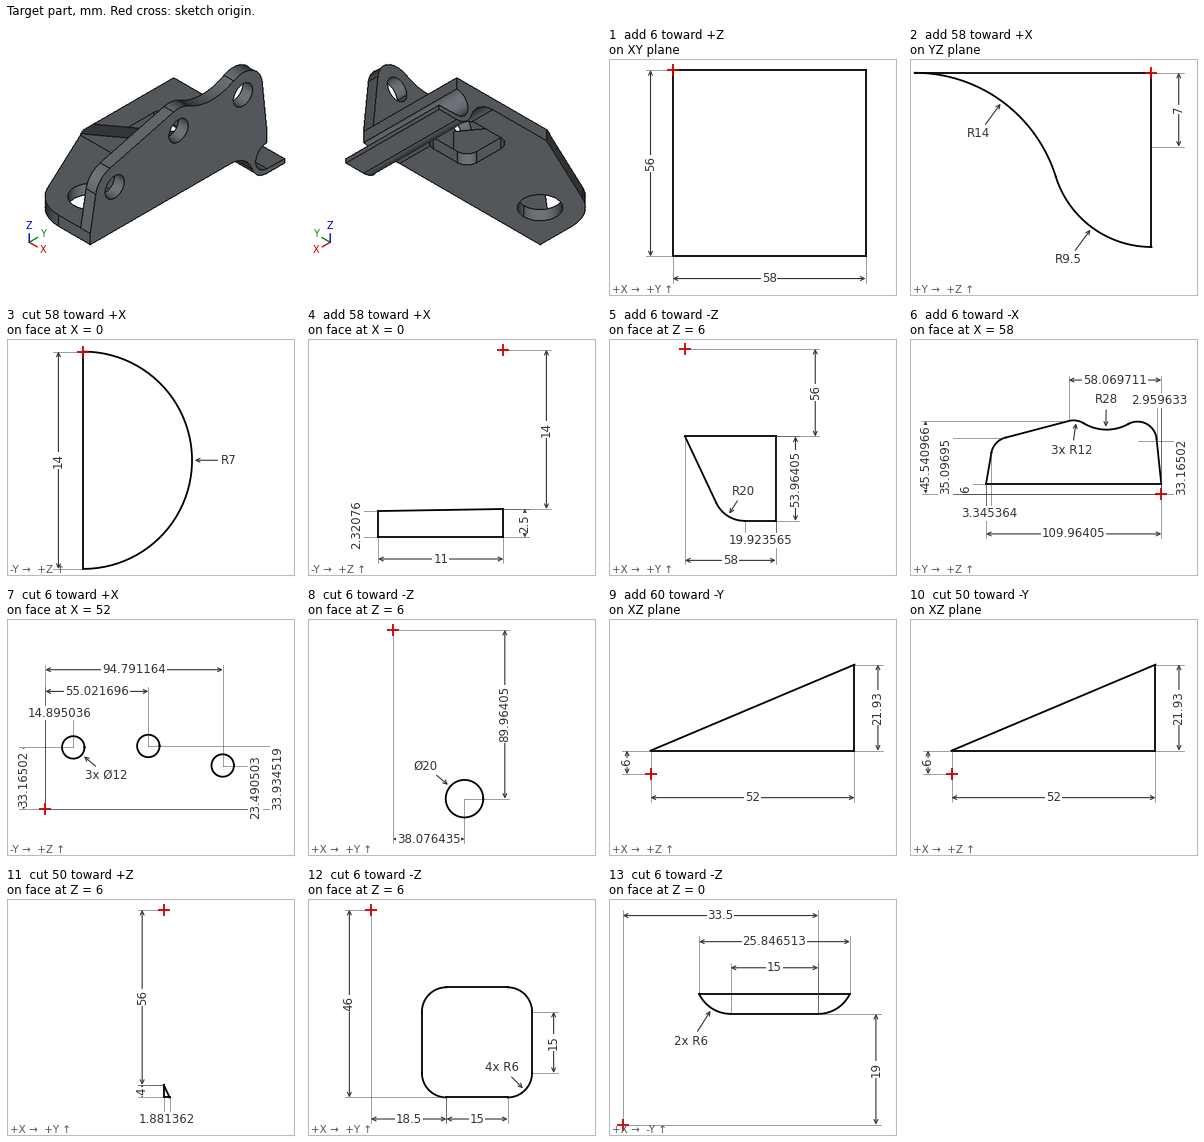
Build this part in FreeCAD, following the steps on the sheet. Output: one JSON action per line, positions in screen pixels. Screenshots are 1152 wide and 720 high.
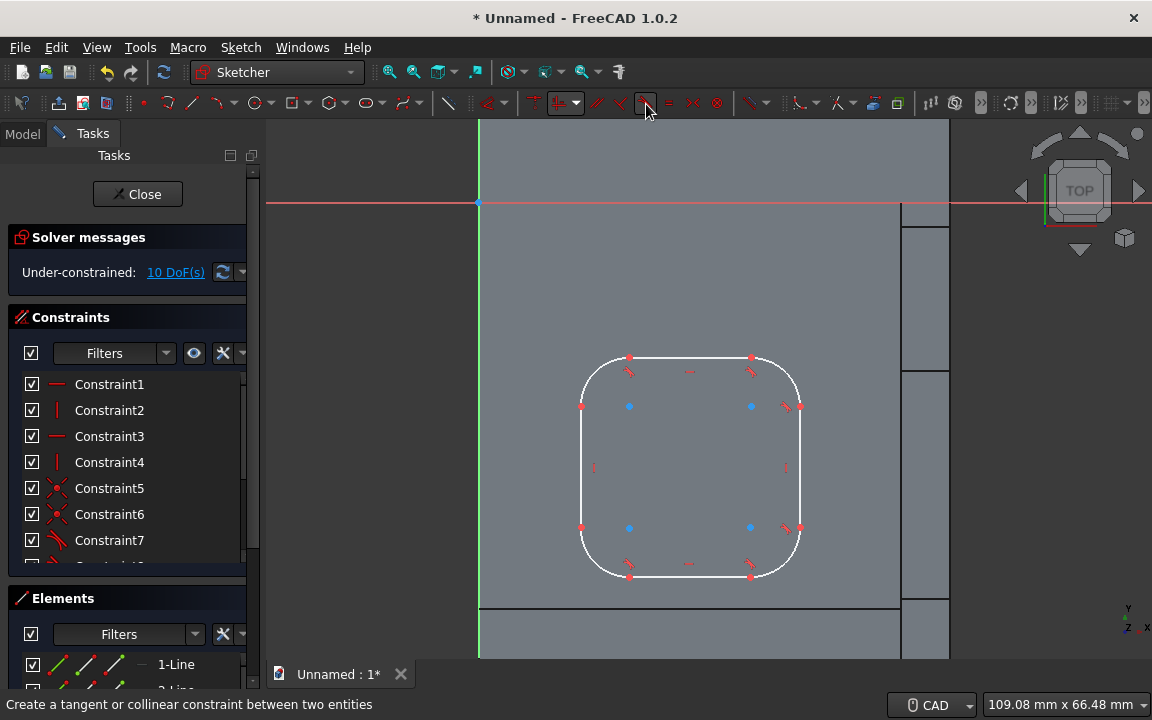
{"action": "left_click", "coordinate": [581, 443]}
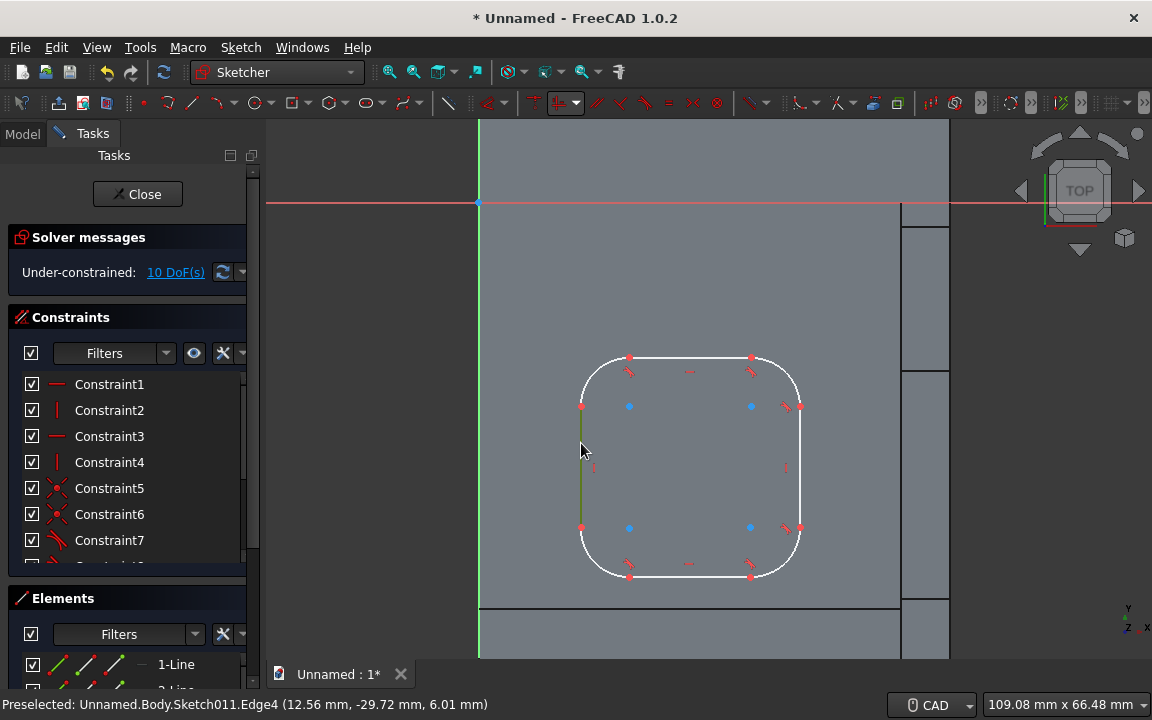
{"action": "left_click", "coordinate": [607, 363]}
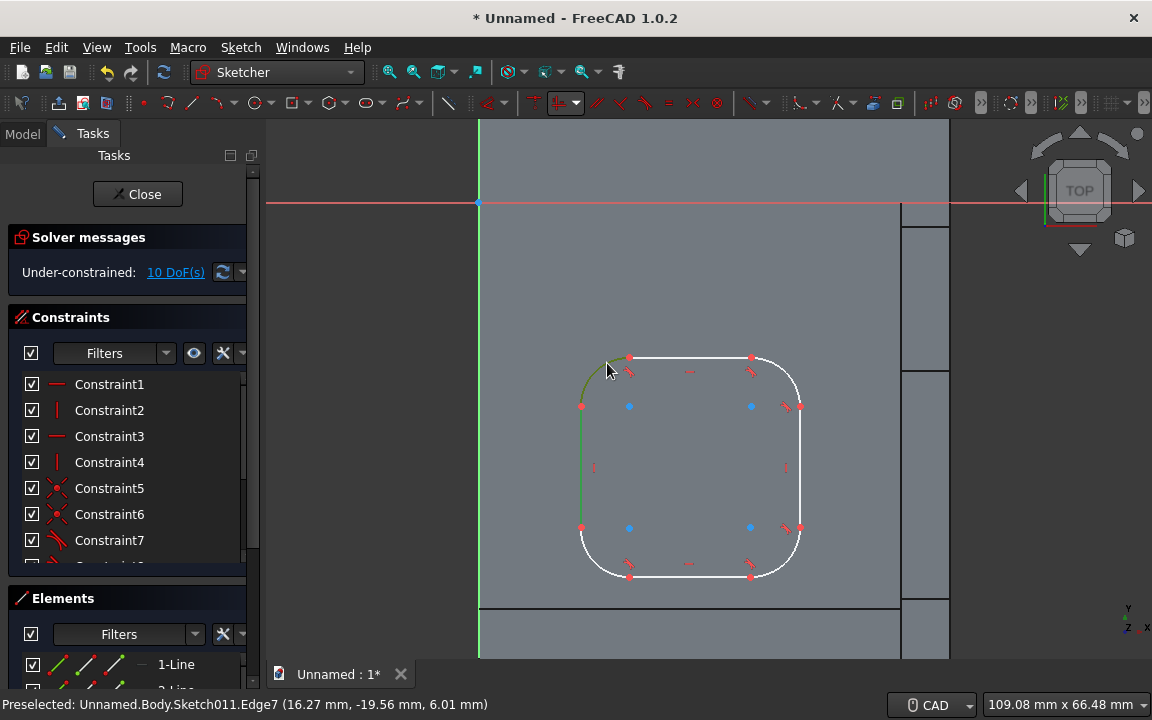
{"action": "left_click", "coordinate": [646, 104]}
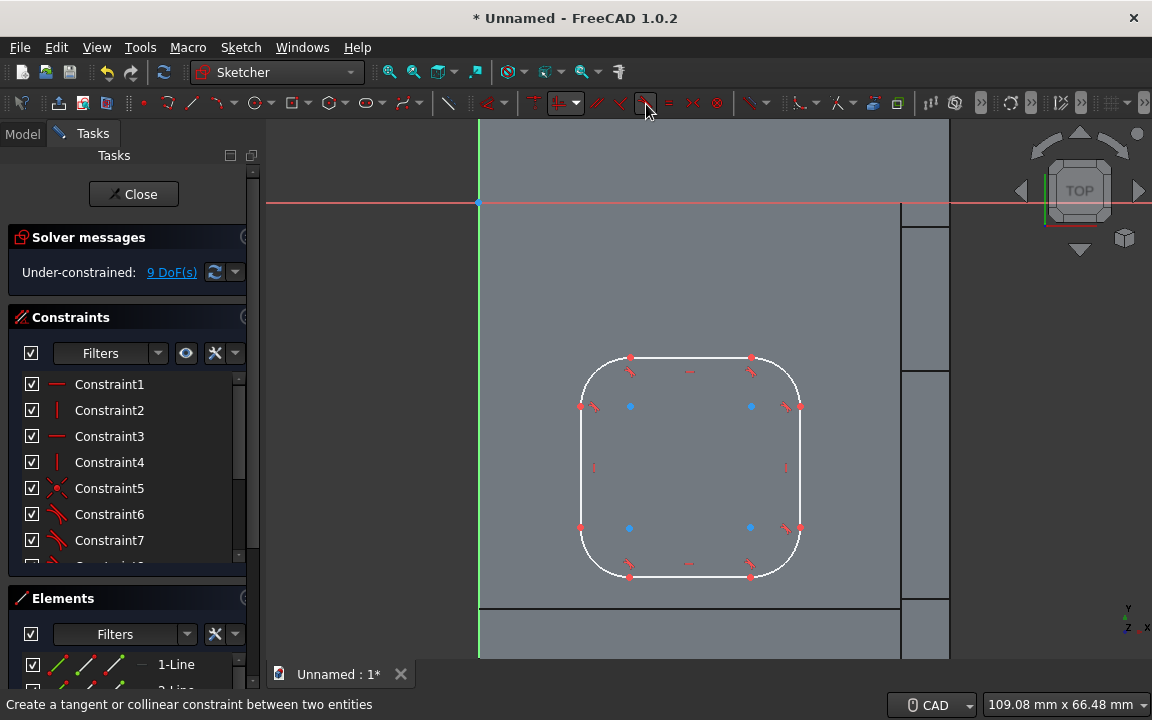
{"action": "left_click", "coordinate": [581, 443]}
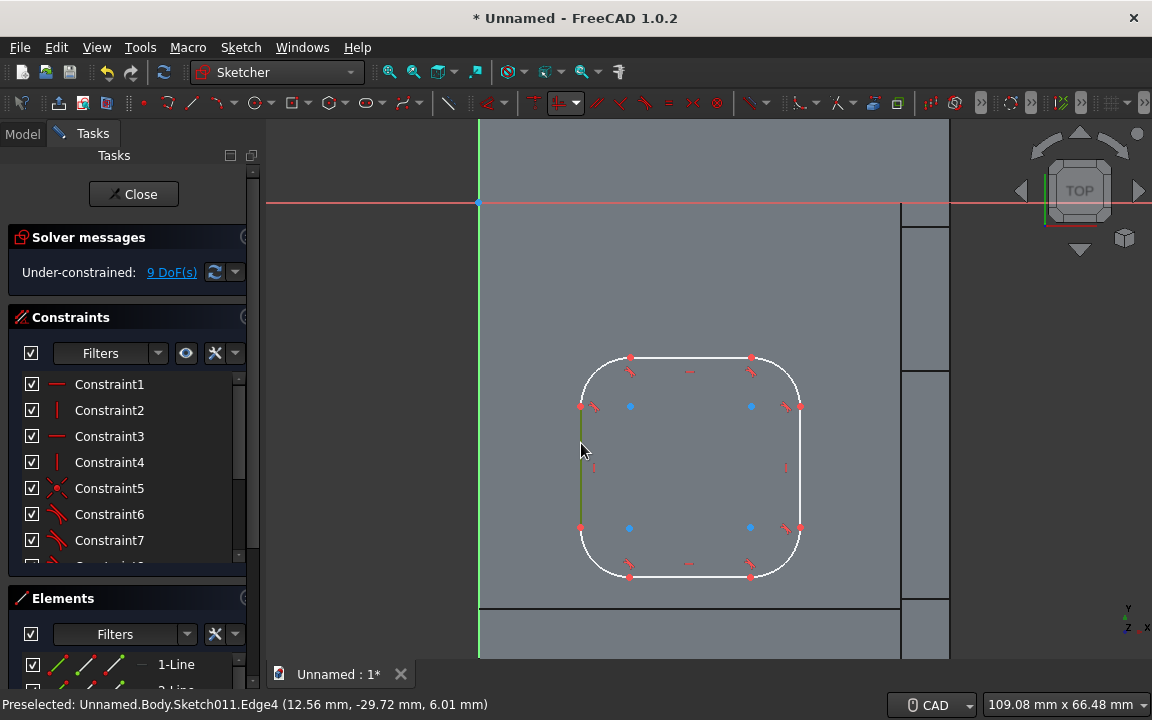
{"action": "left_click", "coordinate": [586, 550]}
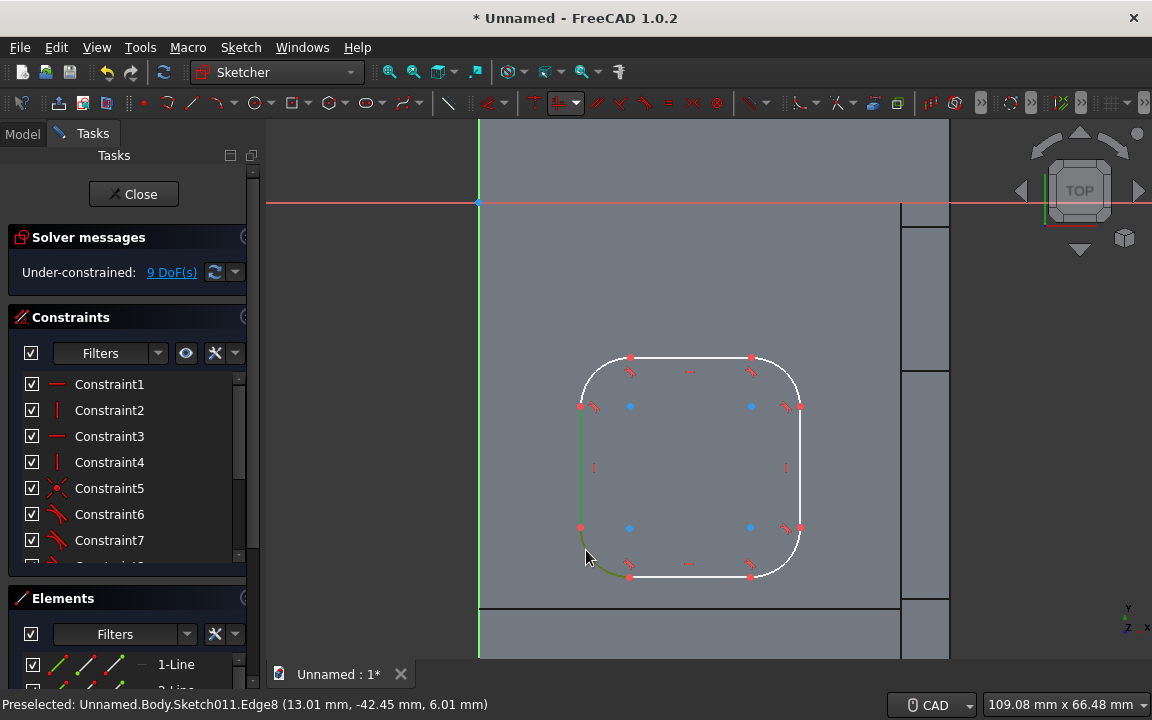
{"action": "left_click", "coordinate": [646, 104]}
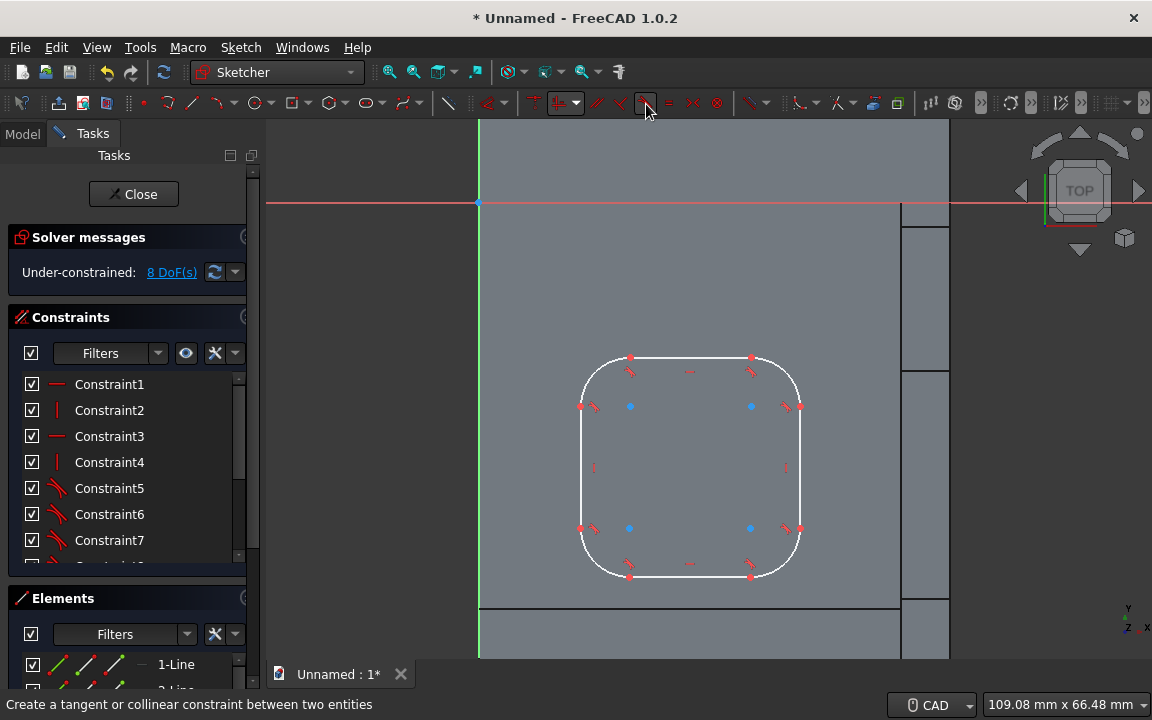
{"action": "left_click", "coordinate": [773, 572]}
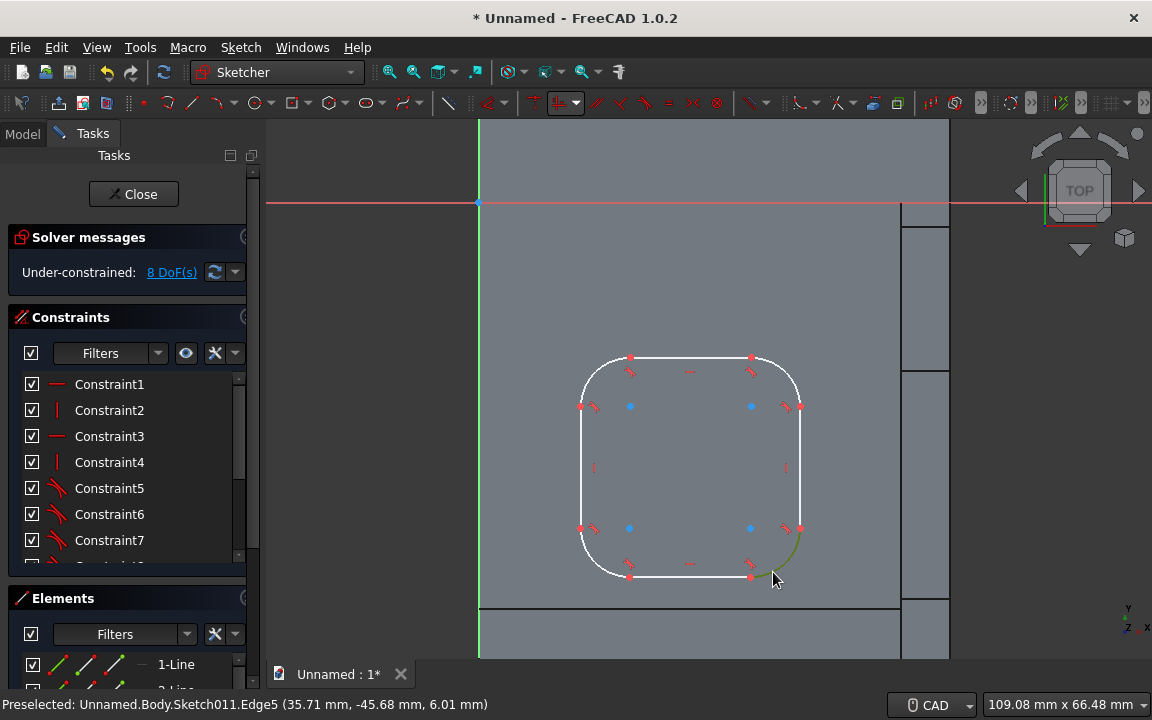
{"action": "left_click", "coordinate": [795, 385]}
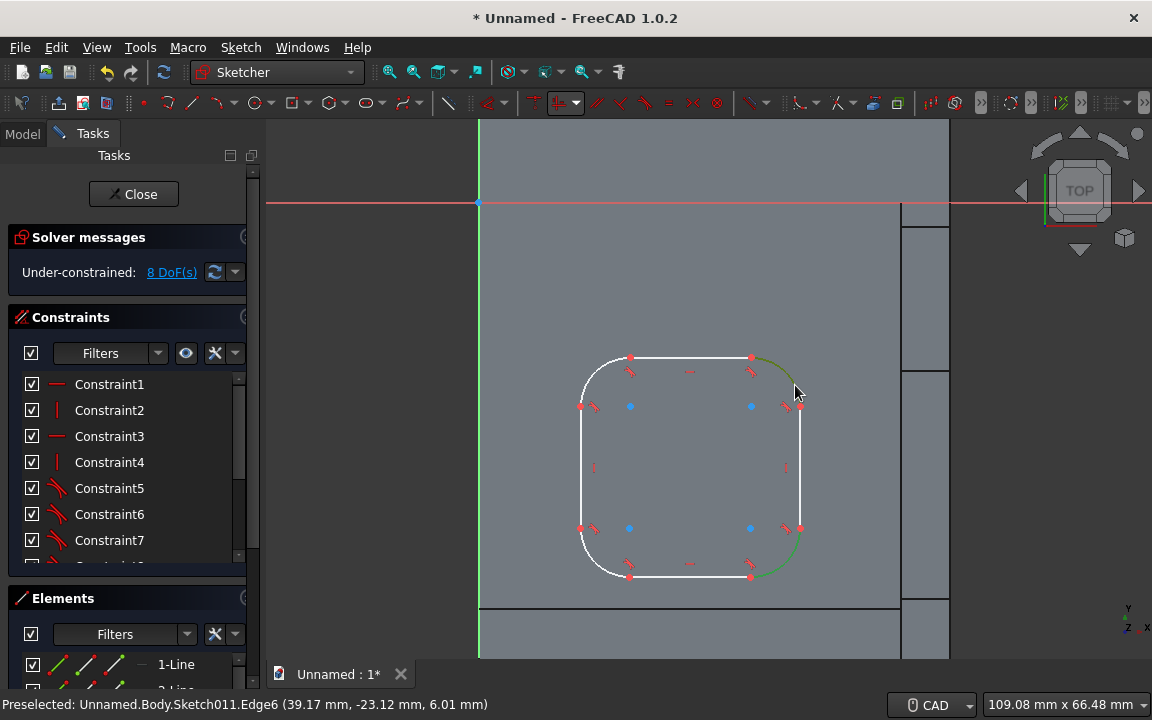
{"action": "left_click", "coordinate": [608, 363]}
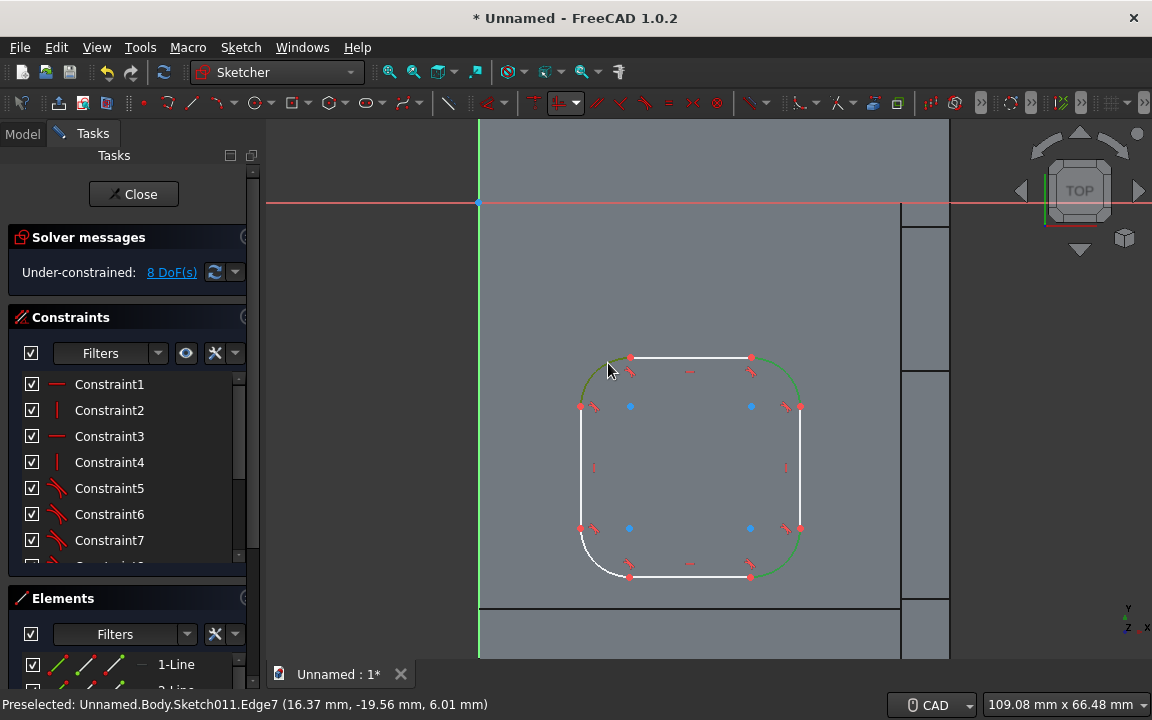
{"action": "left_click", "coordinate": [586, 550]}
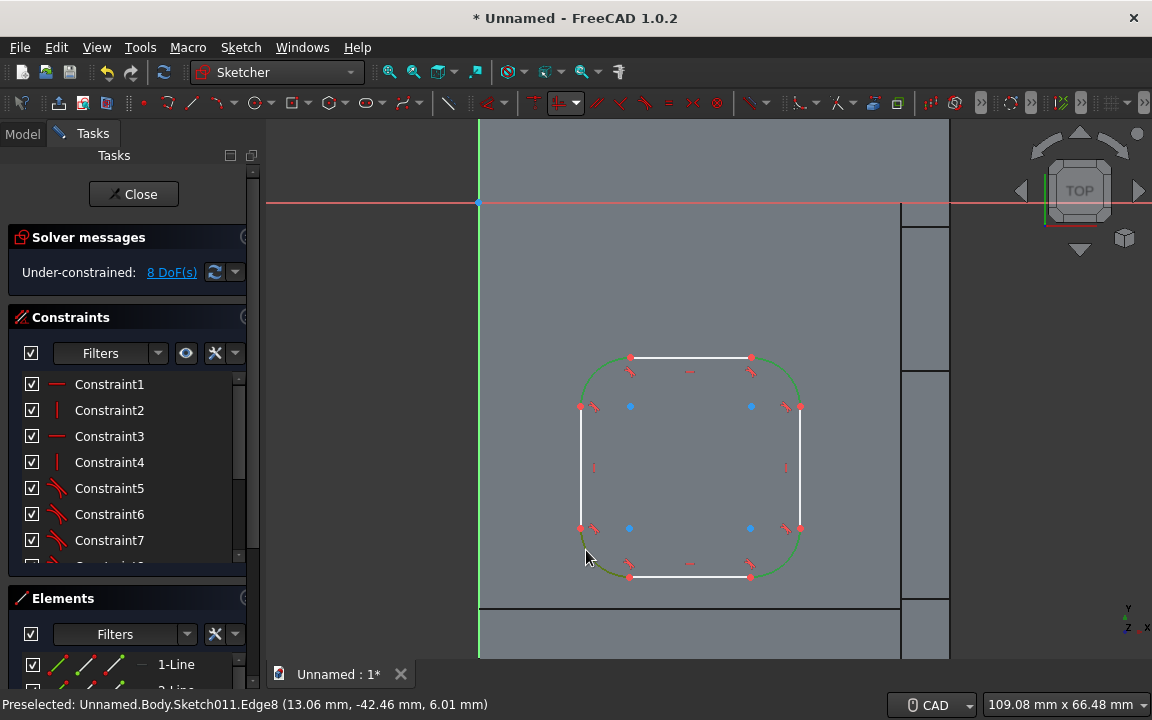
{"action": "left_click", "coordinate": [670, 104]}